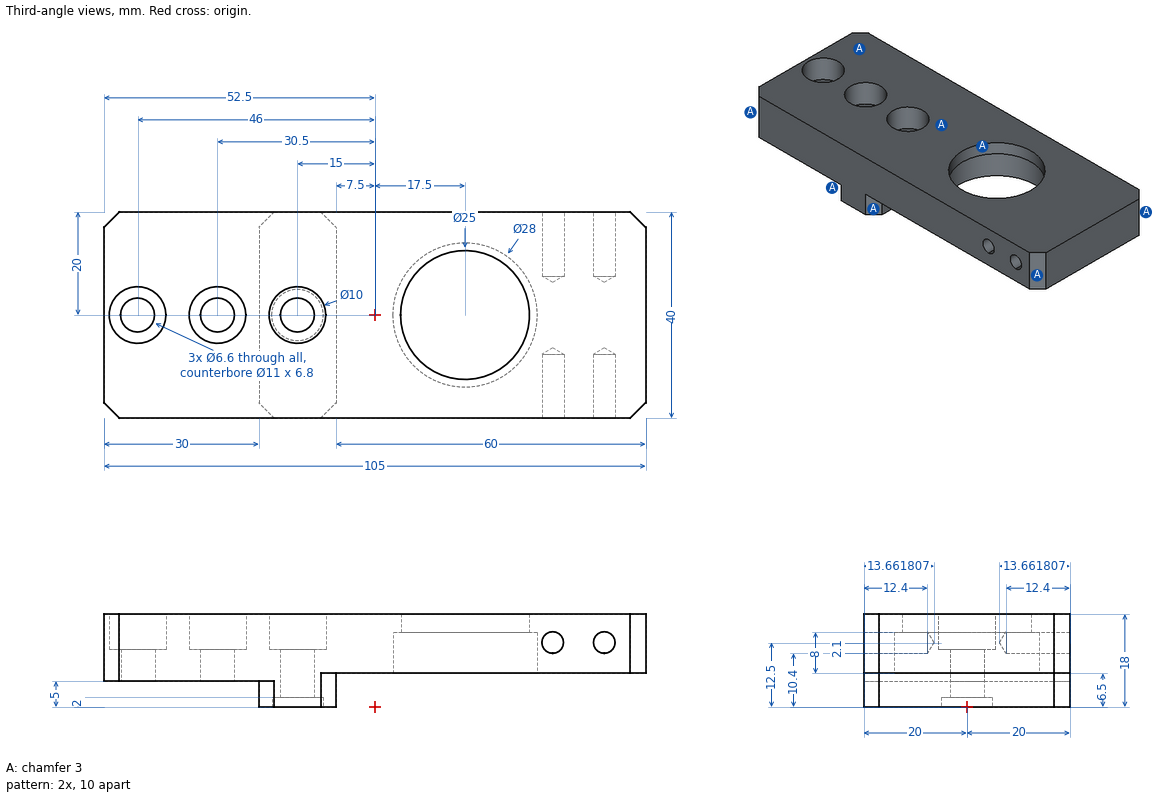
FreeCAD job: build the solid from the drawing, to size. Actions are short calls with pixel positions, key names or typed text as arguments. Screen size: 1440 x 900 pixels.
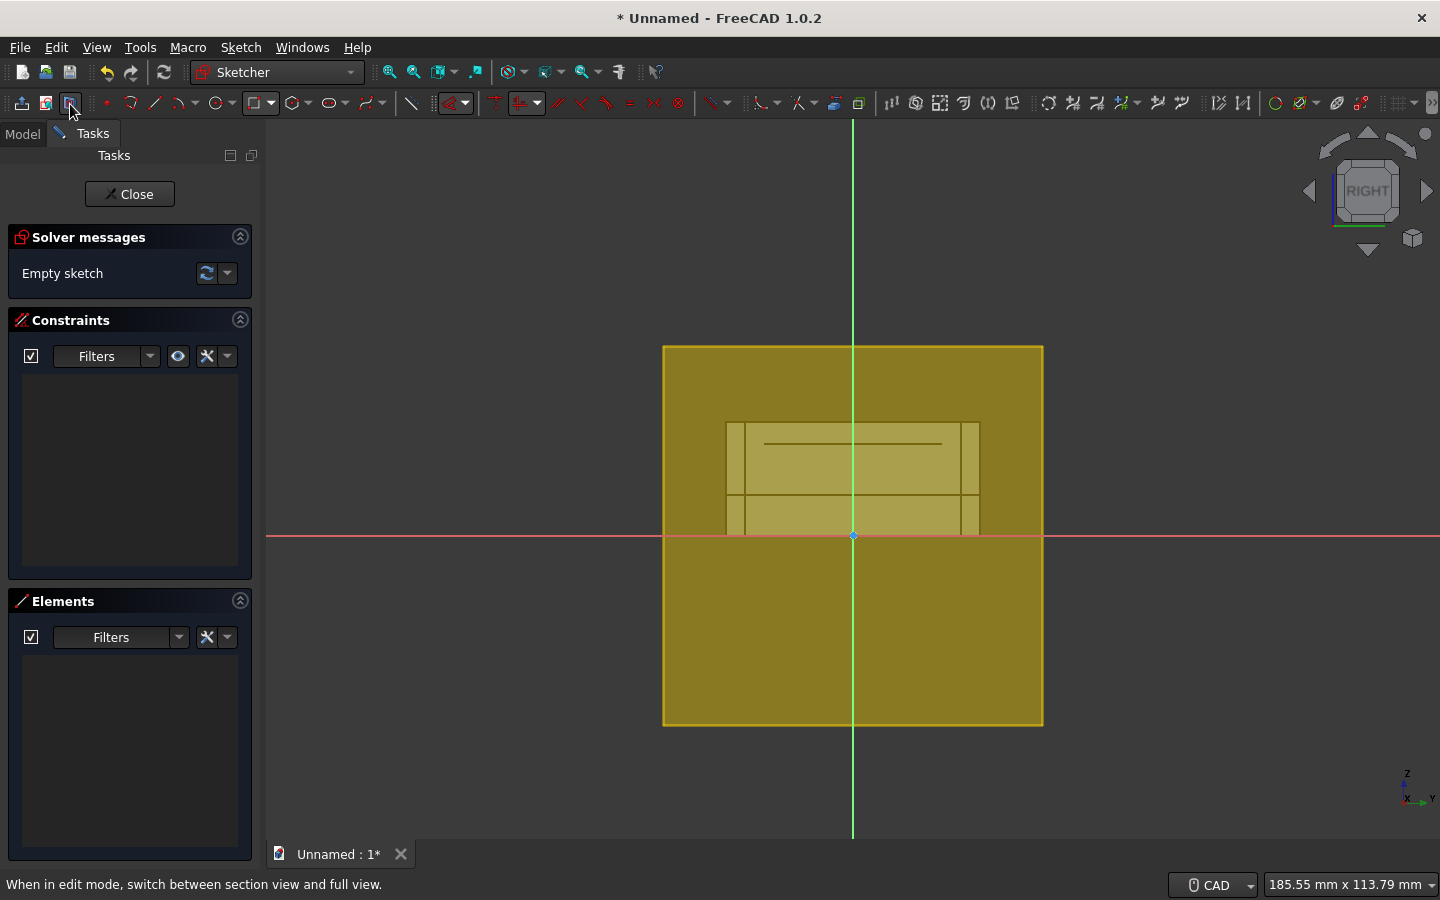
scroll(791, 501, up, 8)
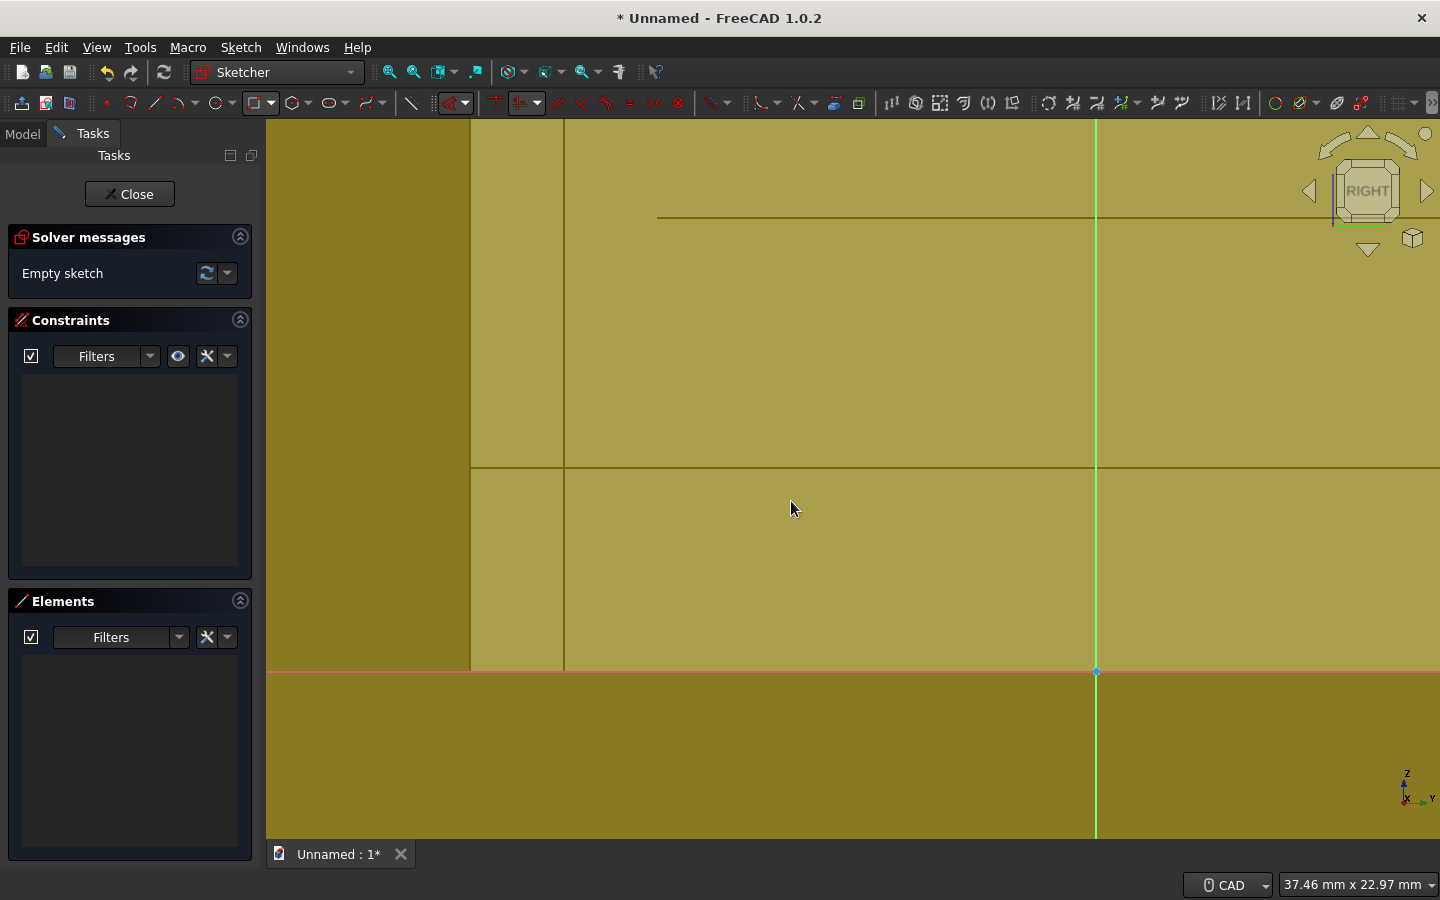
click(132, 104)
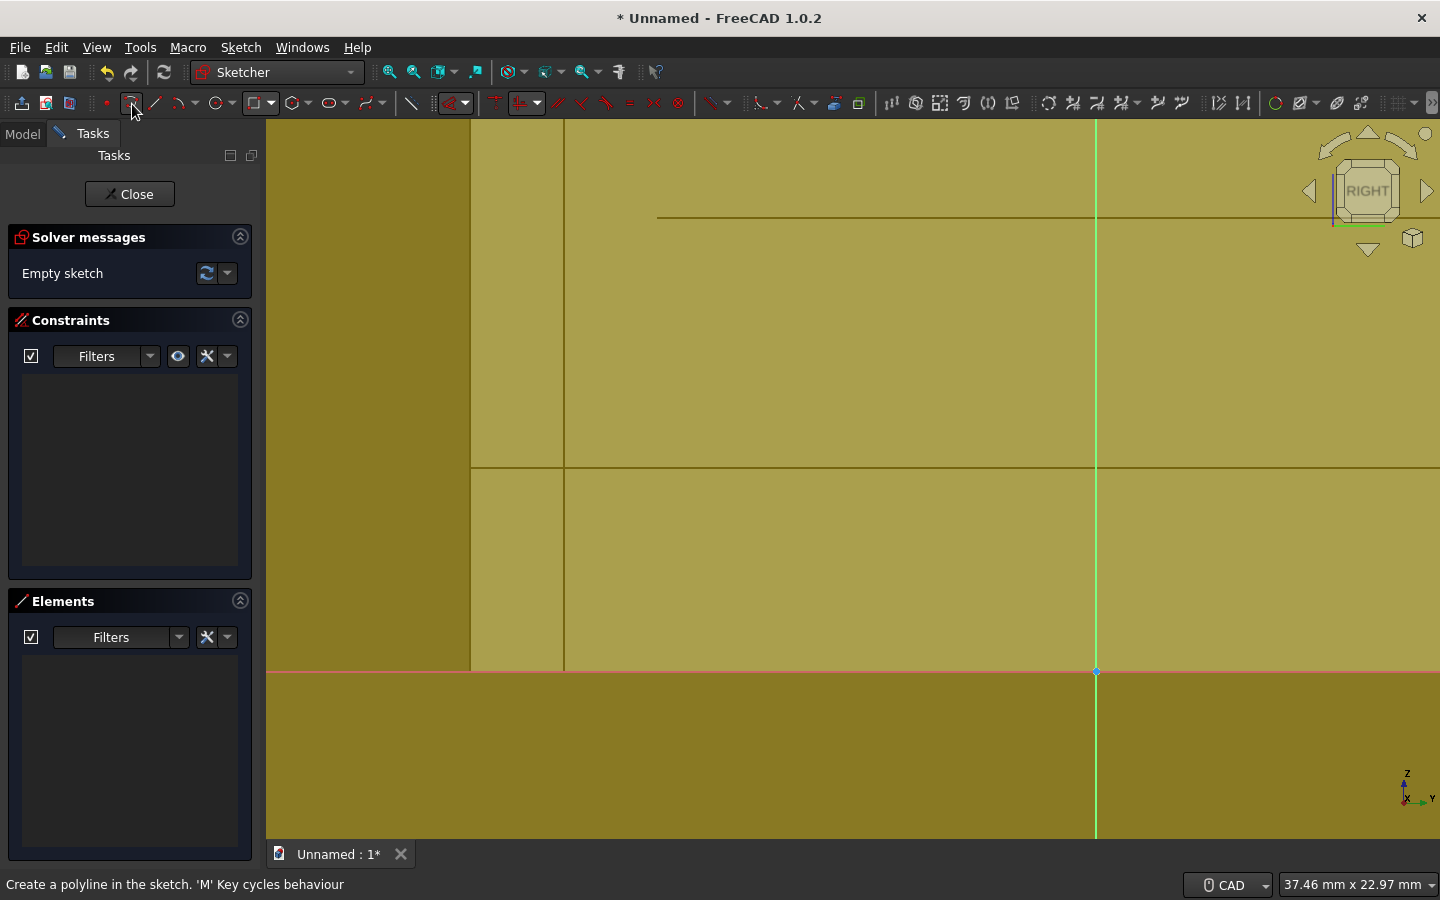
click(858, 346)
click(898, 280)
click(470, 280)
click(470, 346)
click(858, 347)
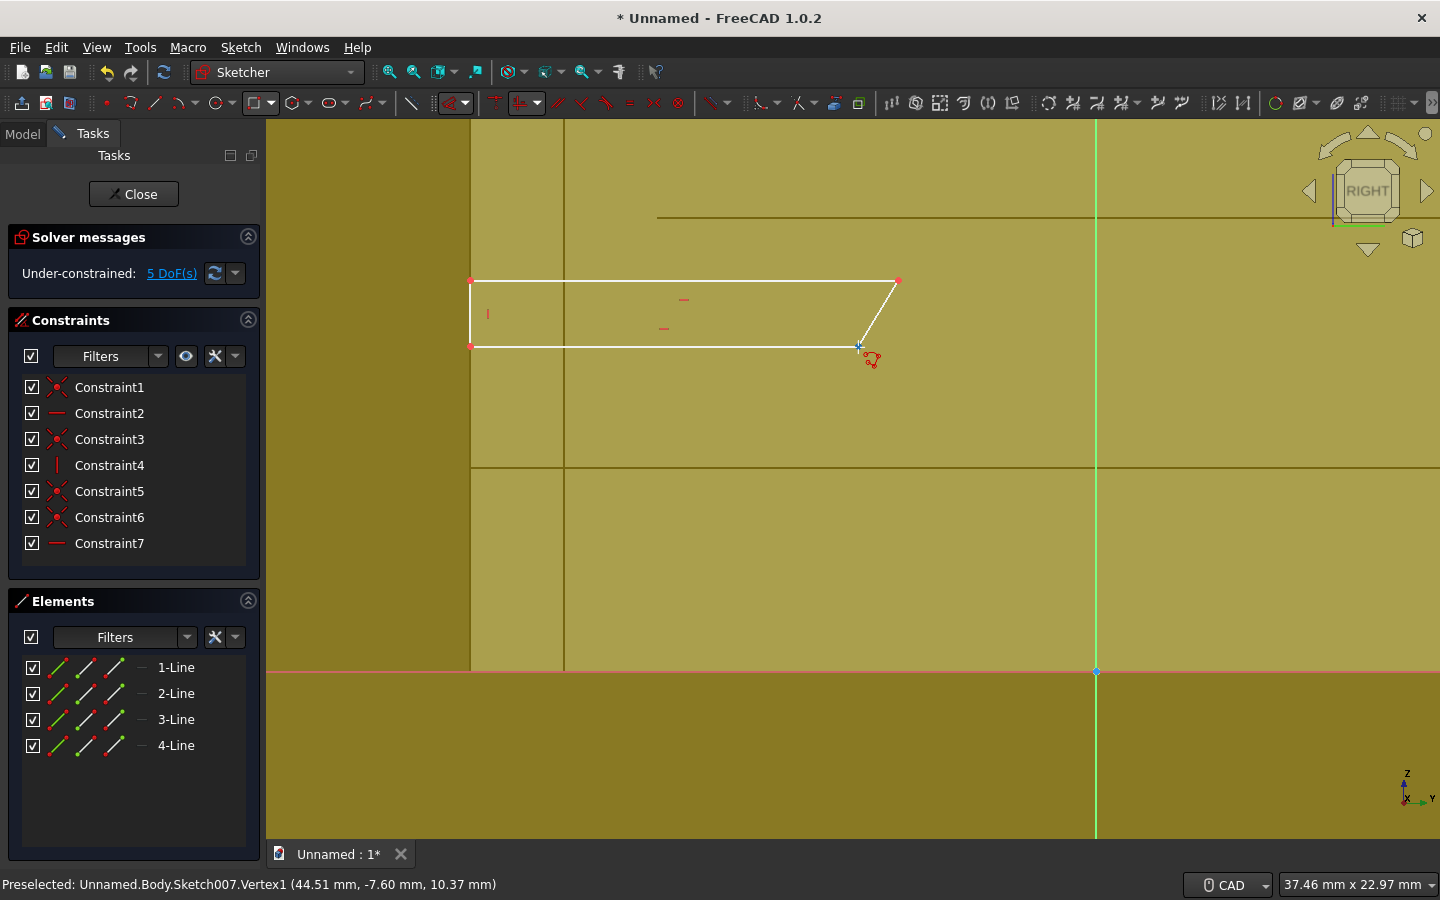
click(156, 104)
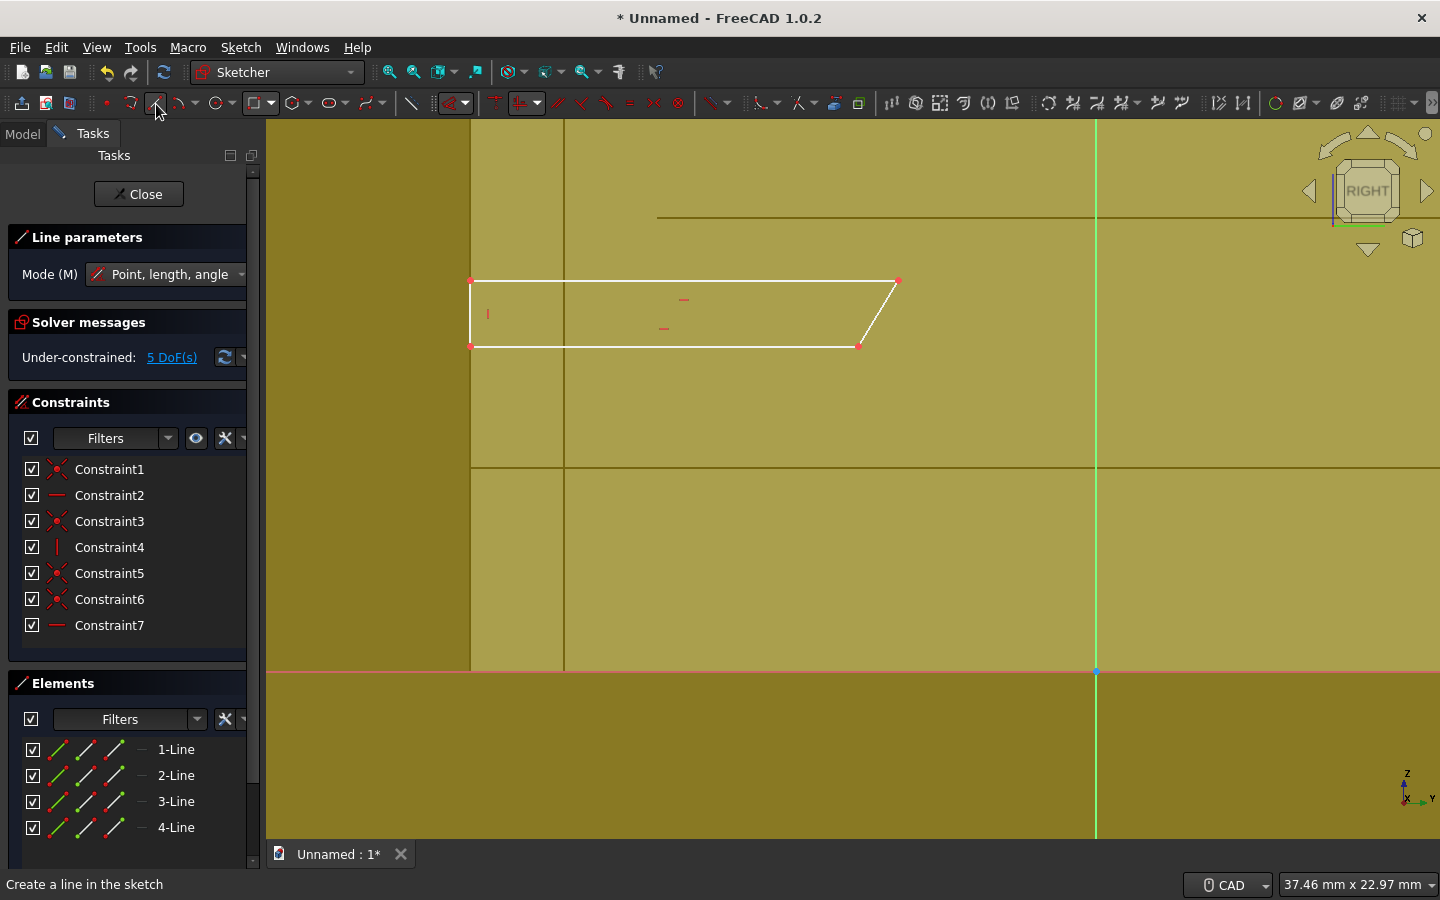
click(941, 280)
click(1069, 280)
key(Escape)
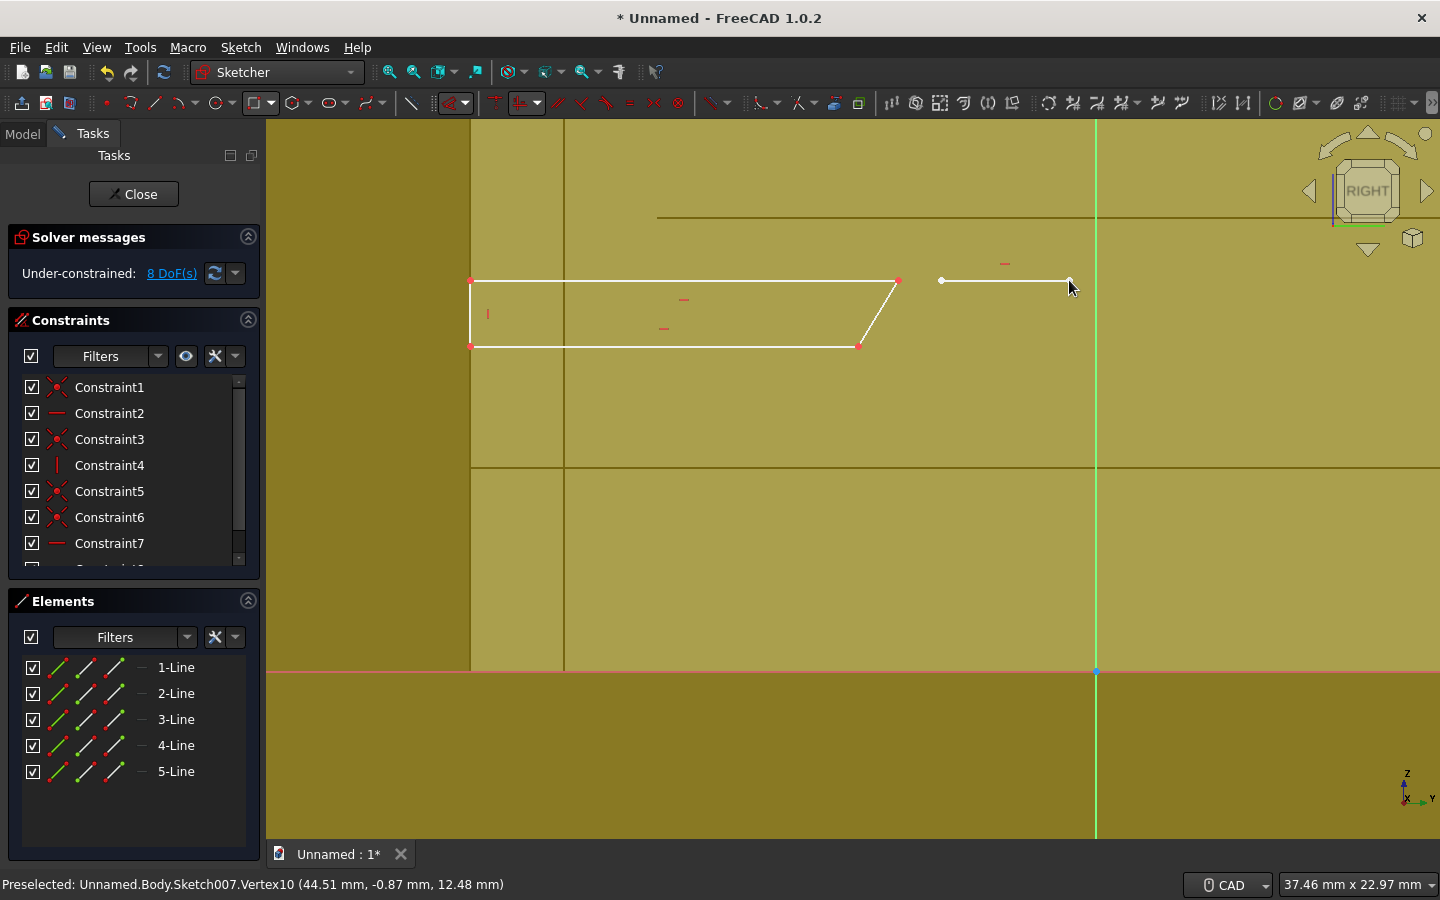
click(979, 281)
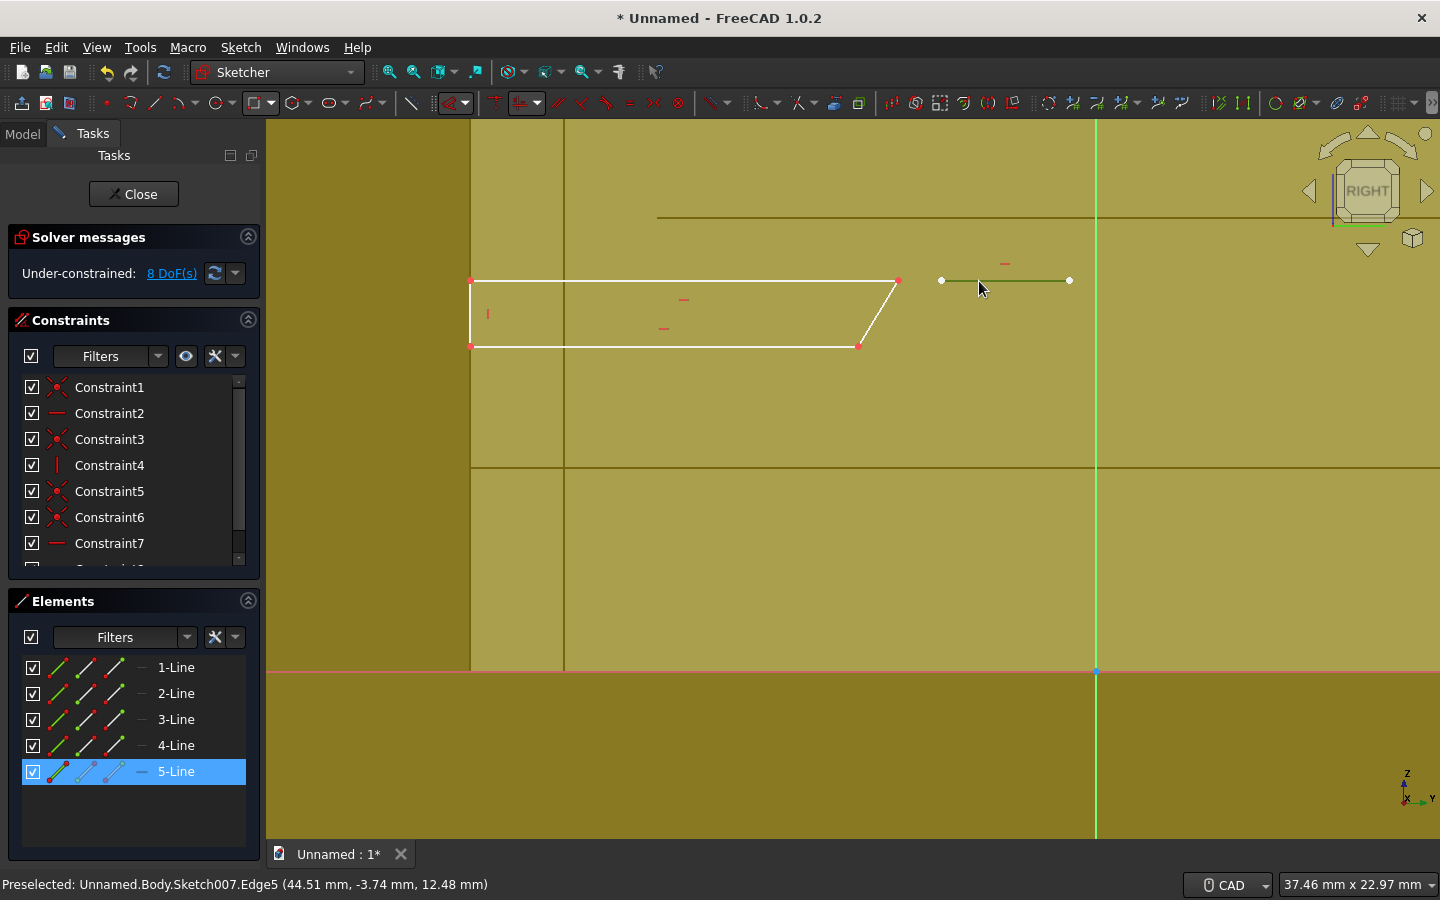
click(412, 104)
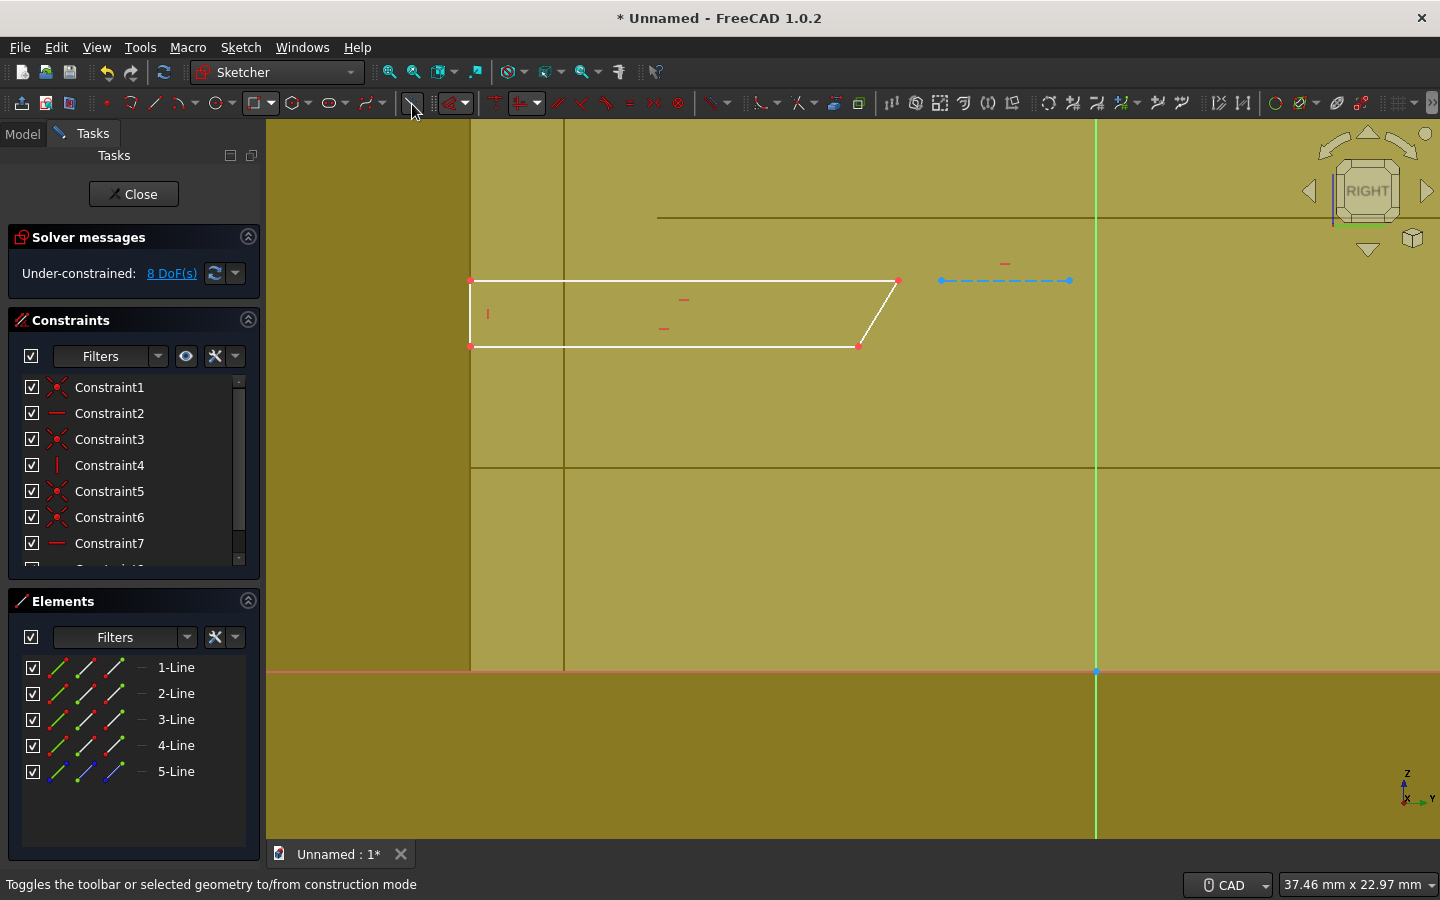
click(470, 301)